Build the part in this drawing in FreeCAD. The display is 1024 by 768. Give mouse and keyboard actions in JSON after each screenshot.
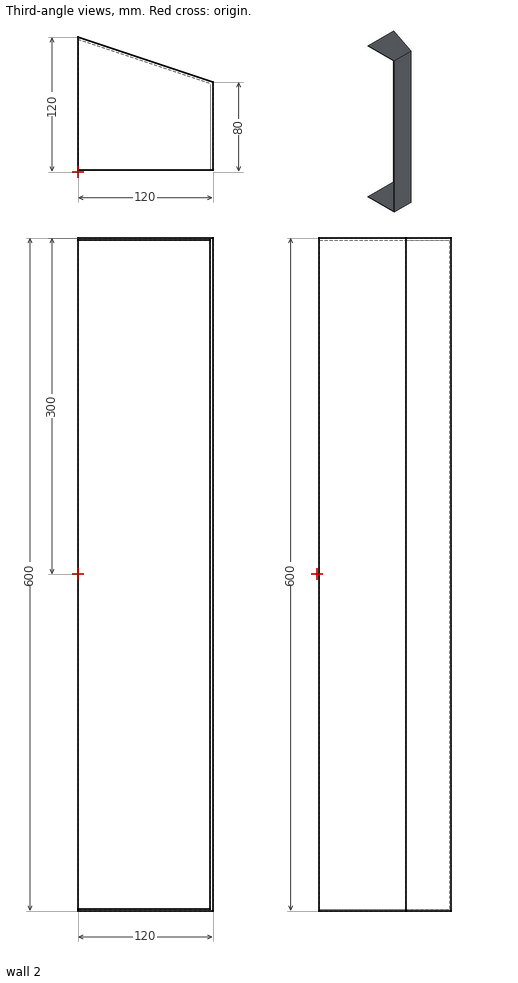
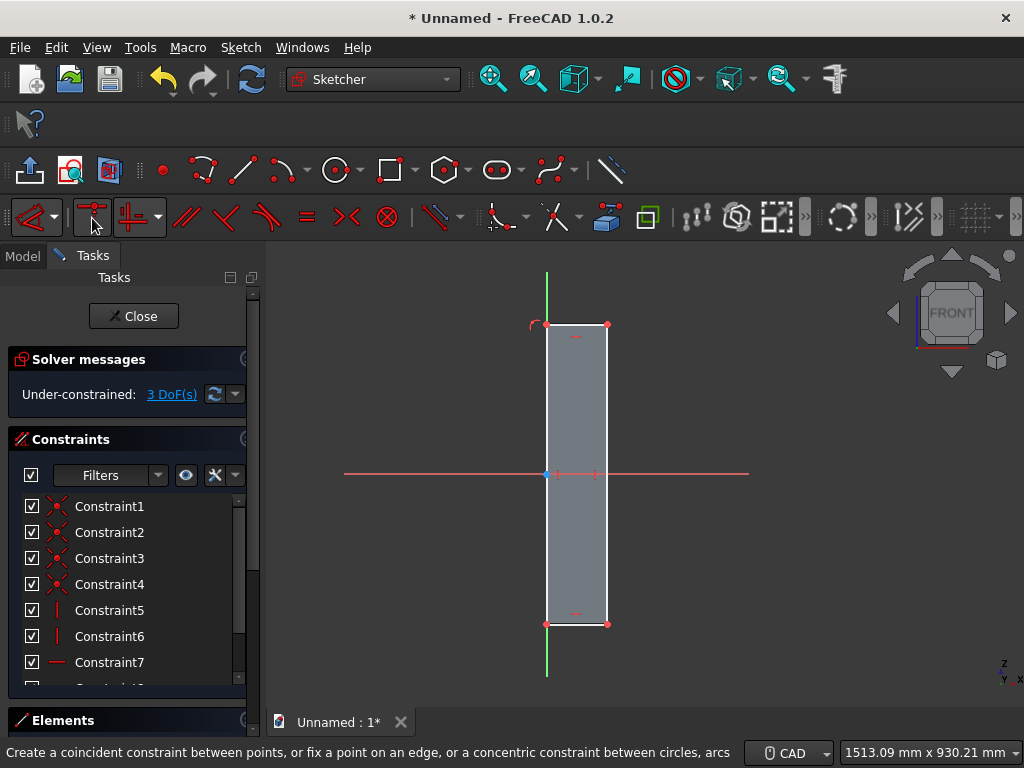
{"action": "left_click", "coordinate": [547, 415]}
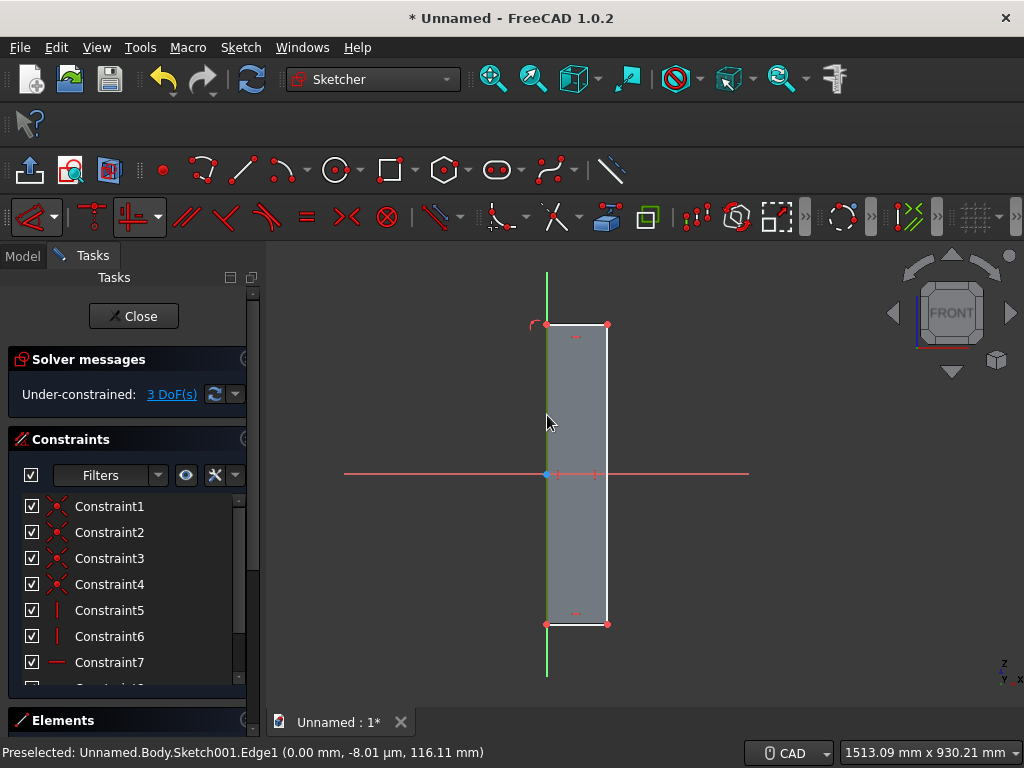
{"action": "left_click", "coordinate": [56, 218]}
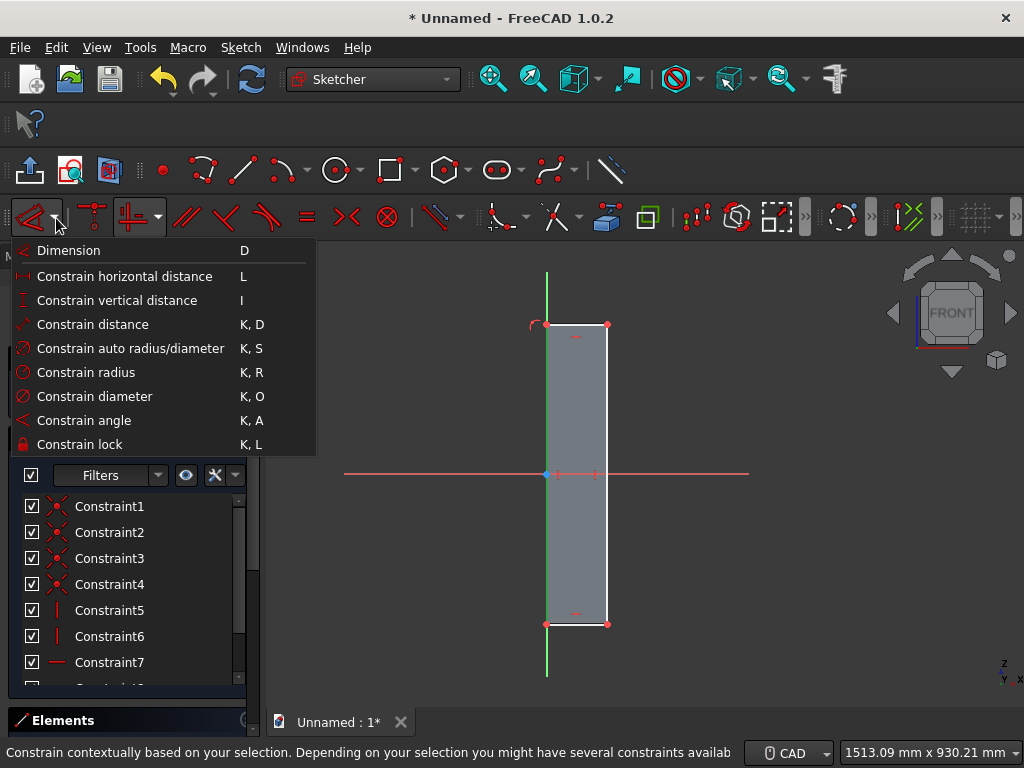
{"action": "left_click", "coordinate": [164, 300]}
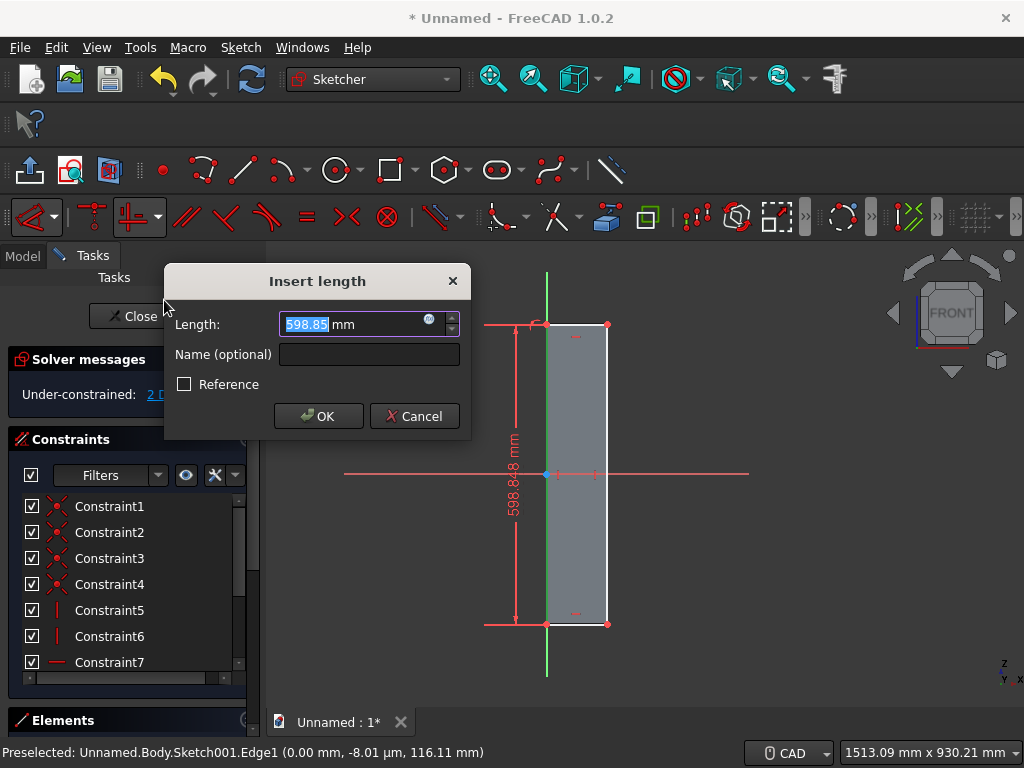
{"action": "type", "text": "600"}
{"action": "key", "text": "Return"}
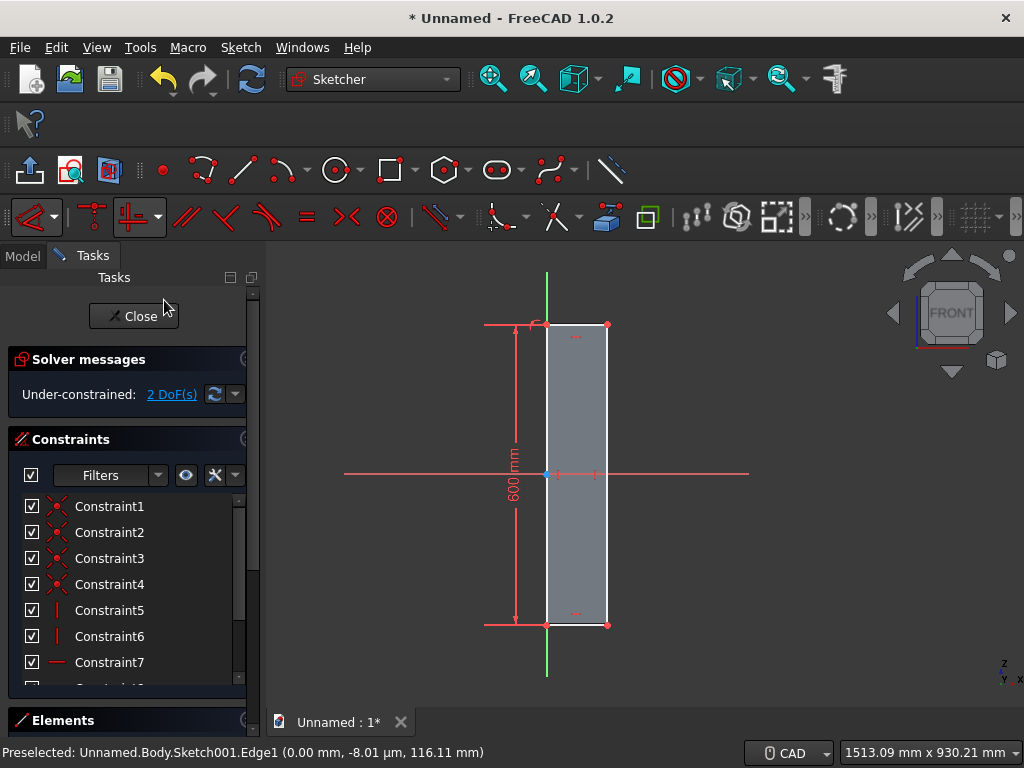
{"action": "left_click", "coordinate": [565, 625]}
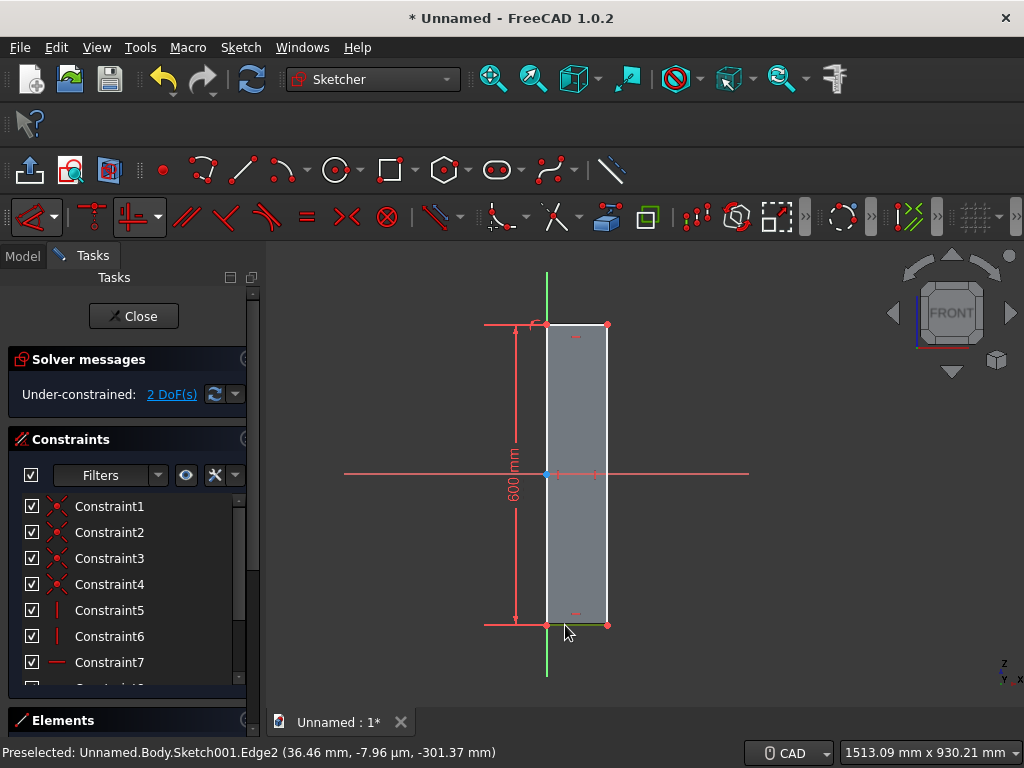
{"action": "key", "text": "l"}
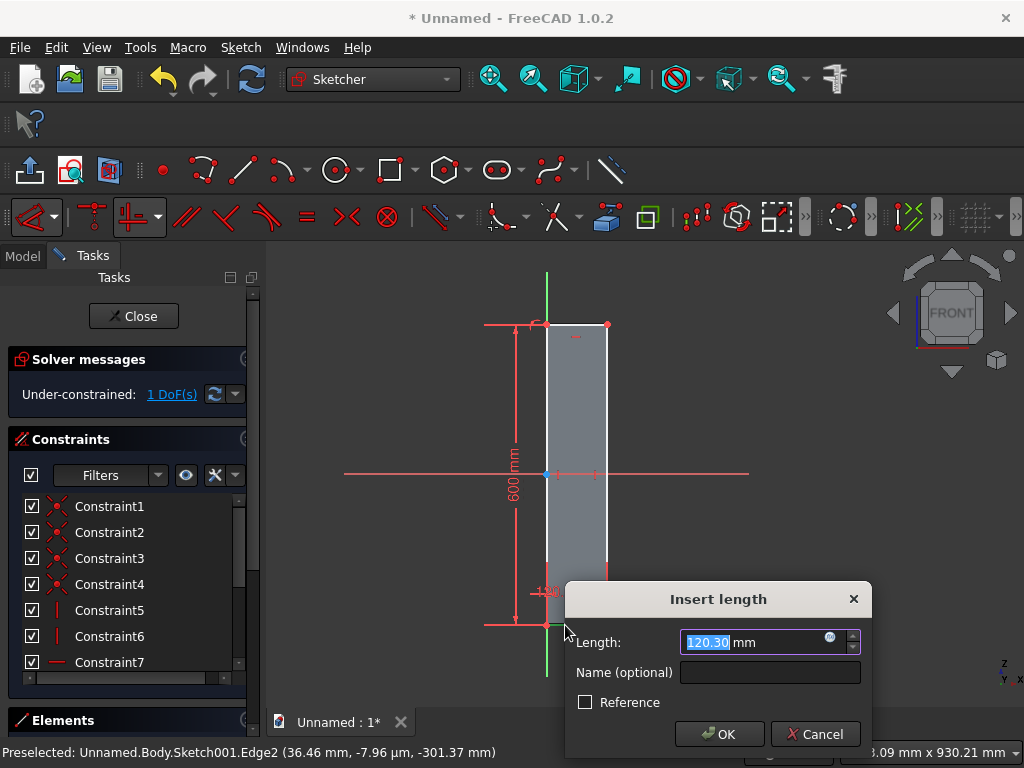
{"action": "type", "text": "120"}
{"action": "key", "text": "Return"}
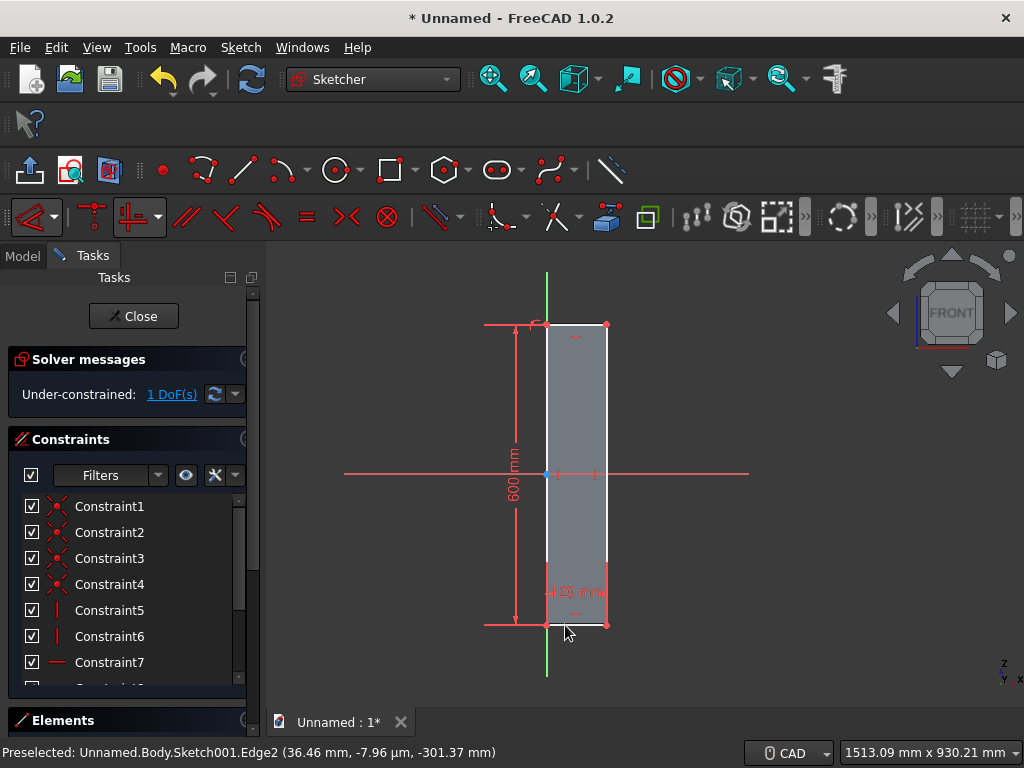
{"action": "left_click", "coordinate": [547, 325]}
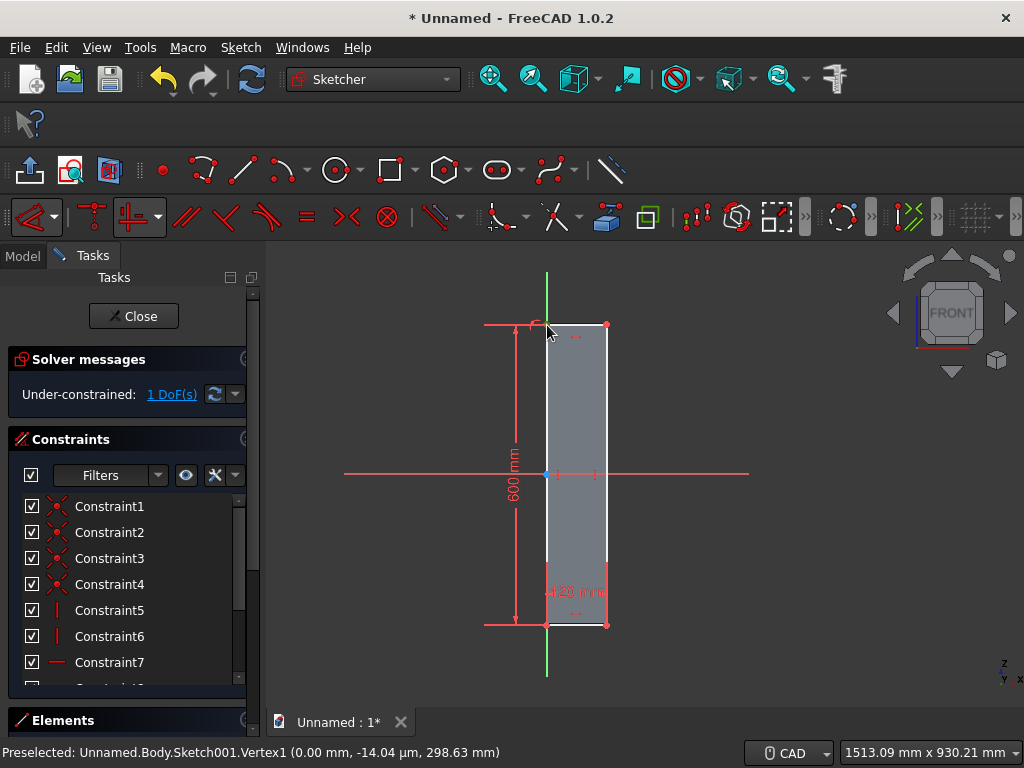
{"action": "left_click", "coordinate": [56, 218]}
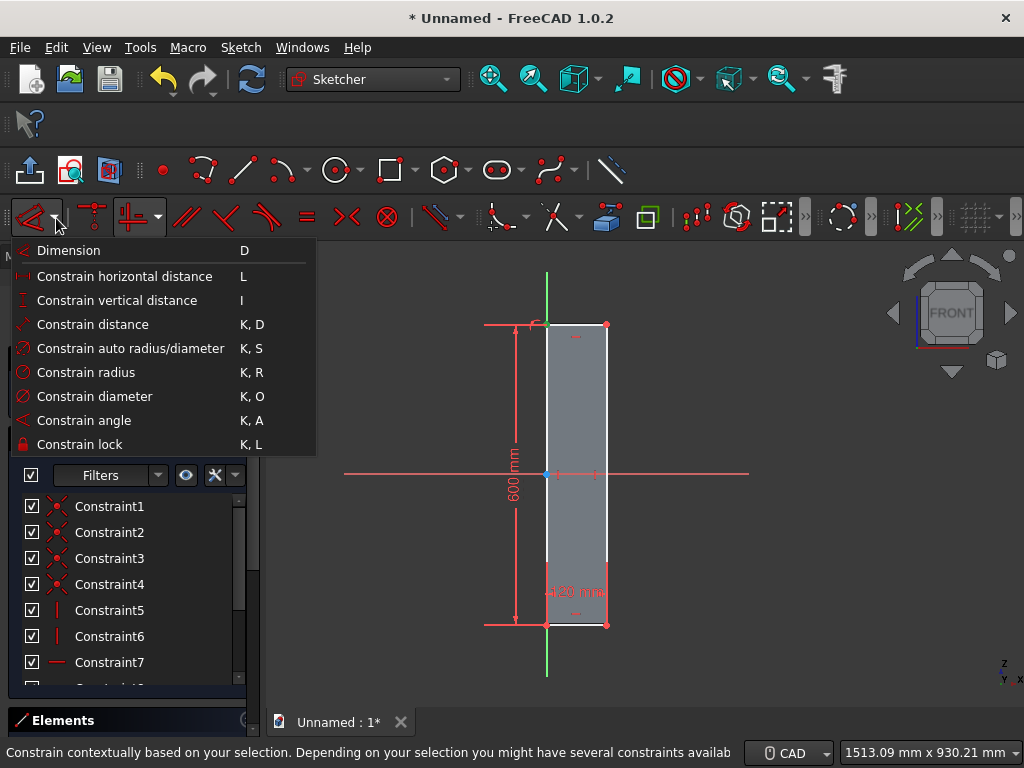
{"action": "left_click", "coordinate": [164, 300]}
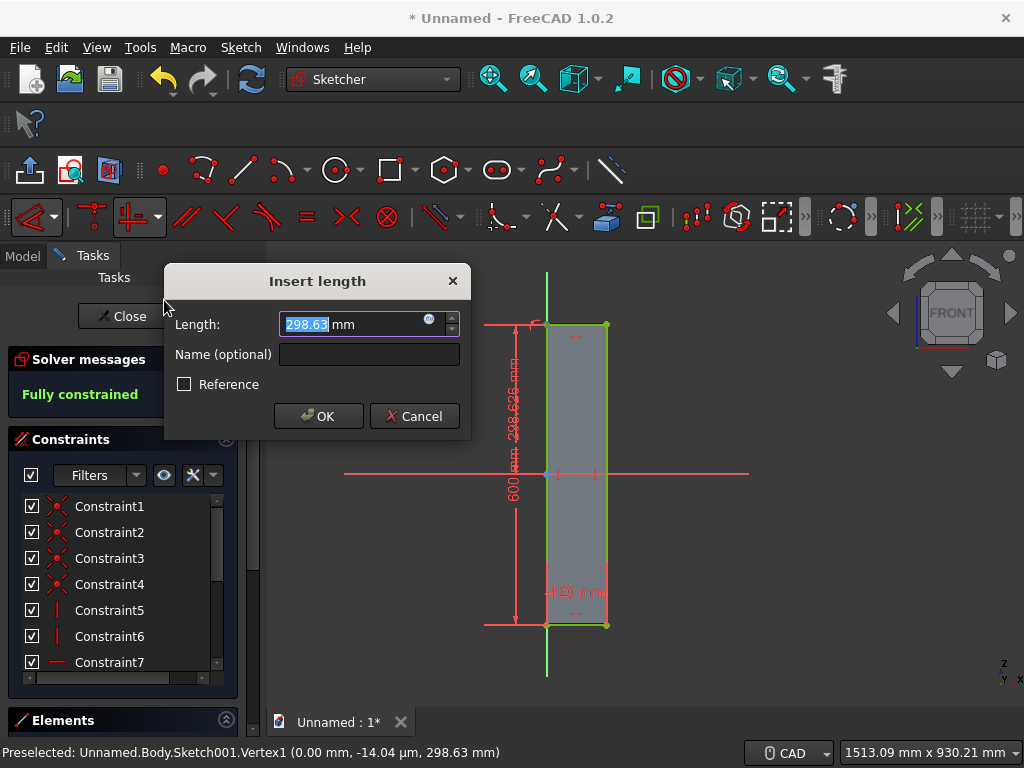
{"action": "type", "text": "300"}
{"action": "key", "text": "Return"}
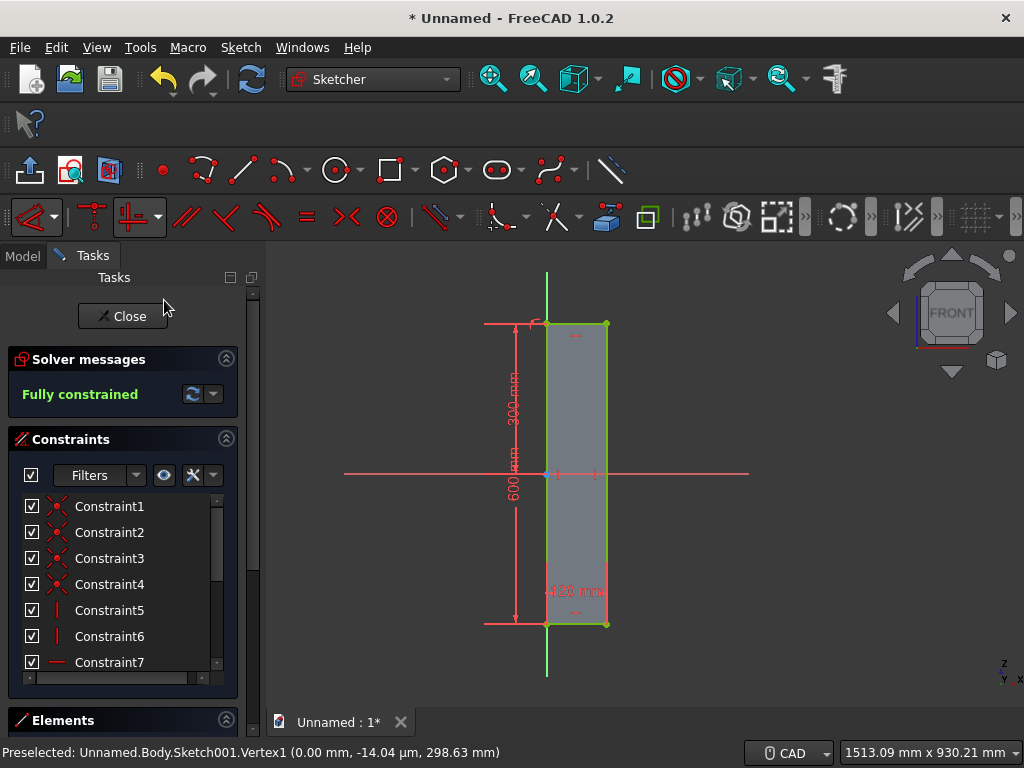
{"action": "left_click", "coordinate": [123, 316]}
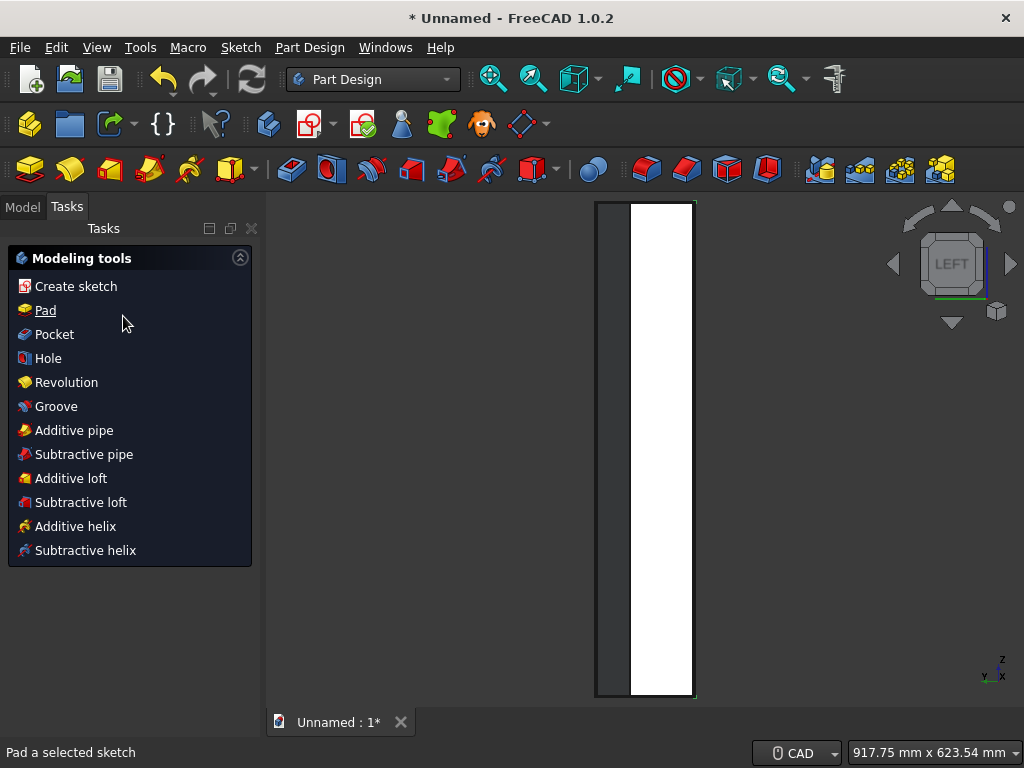
{"action": "left_click", "coordinate": [292, 170]}